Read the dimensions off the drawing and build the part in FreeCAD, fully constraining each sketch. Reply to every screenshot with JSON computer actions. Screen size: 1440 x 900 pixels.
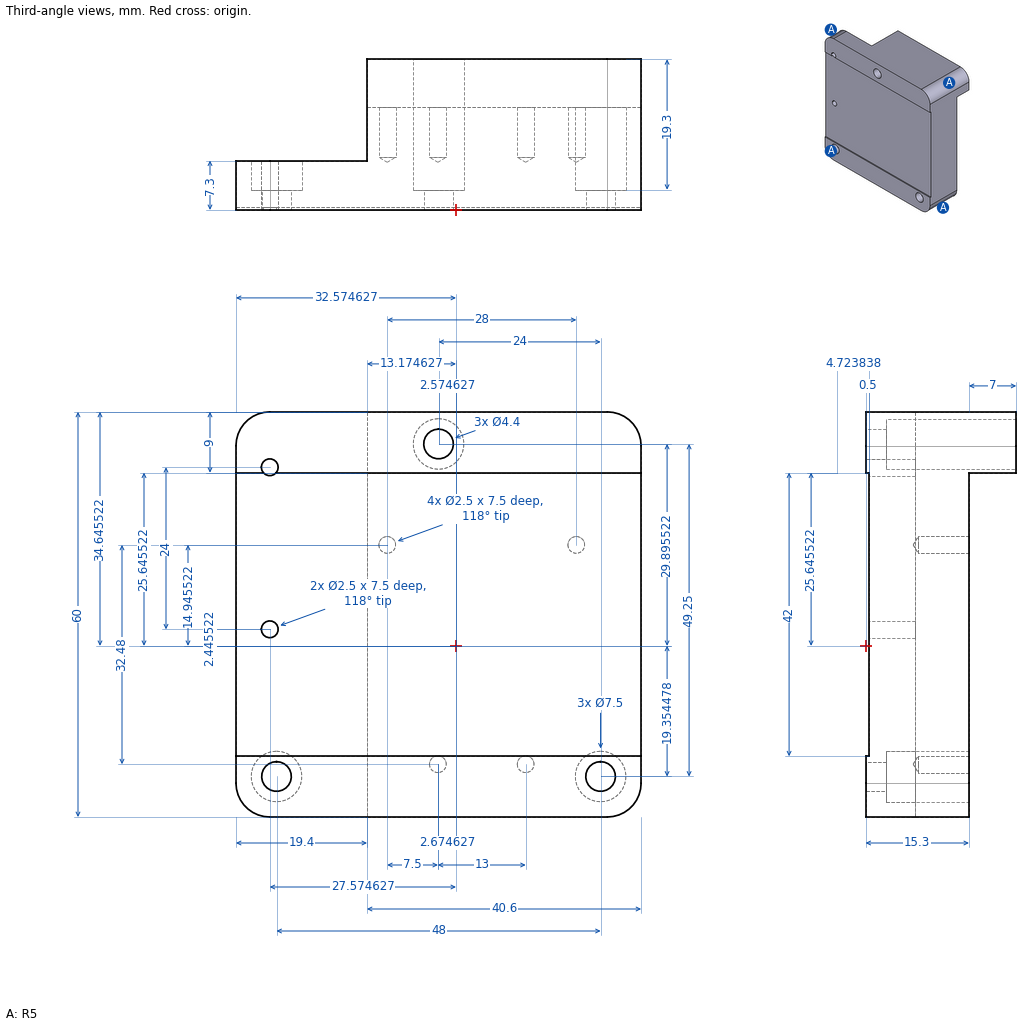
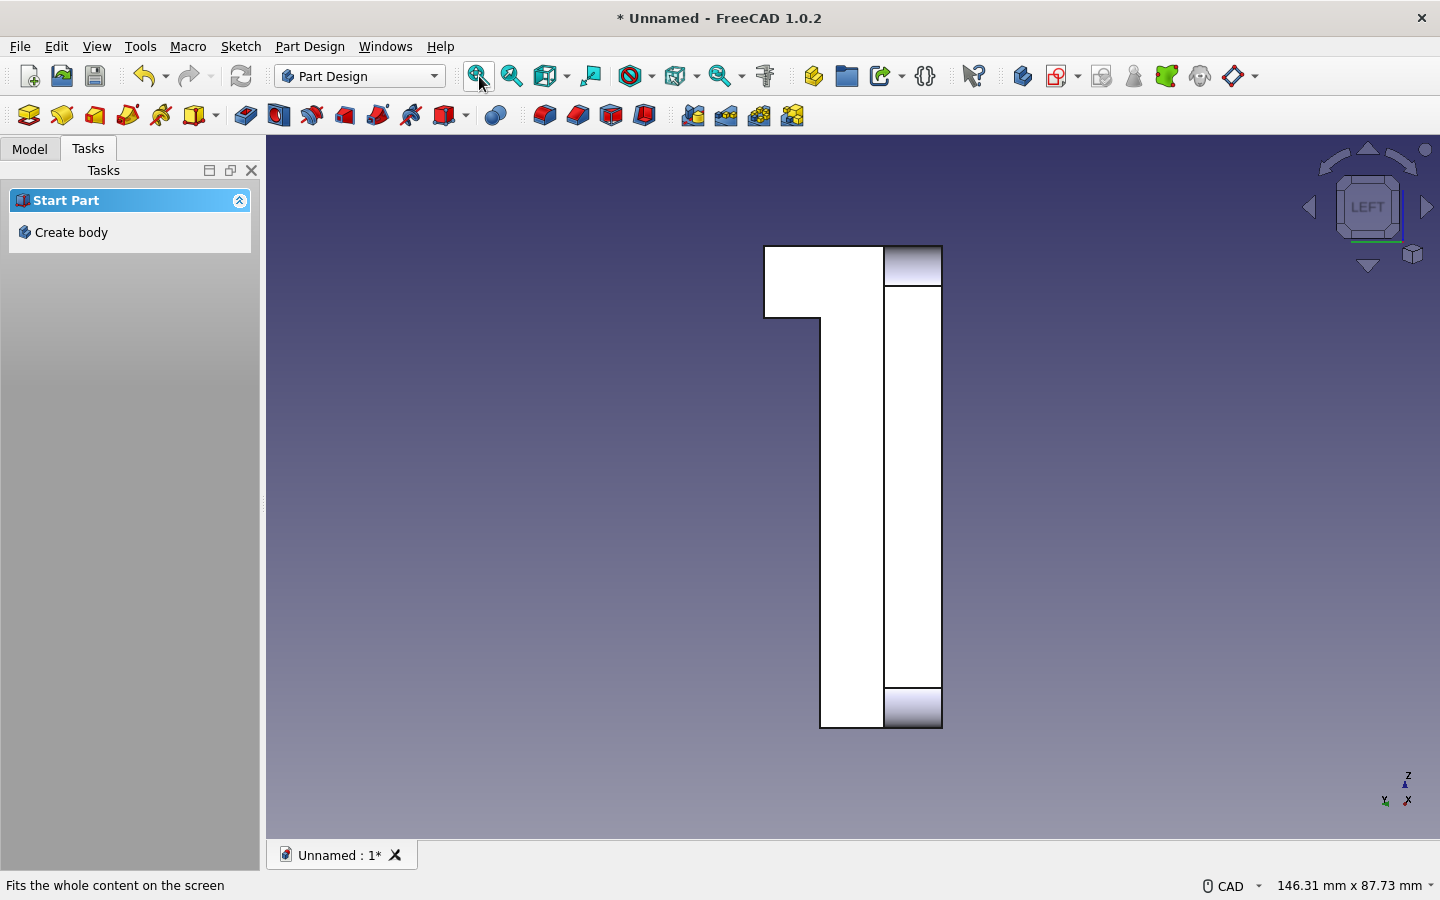
{"action": "left_click", "coordinate": [913, 543]}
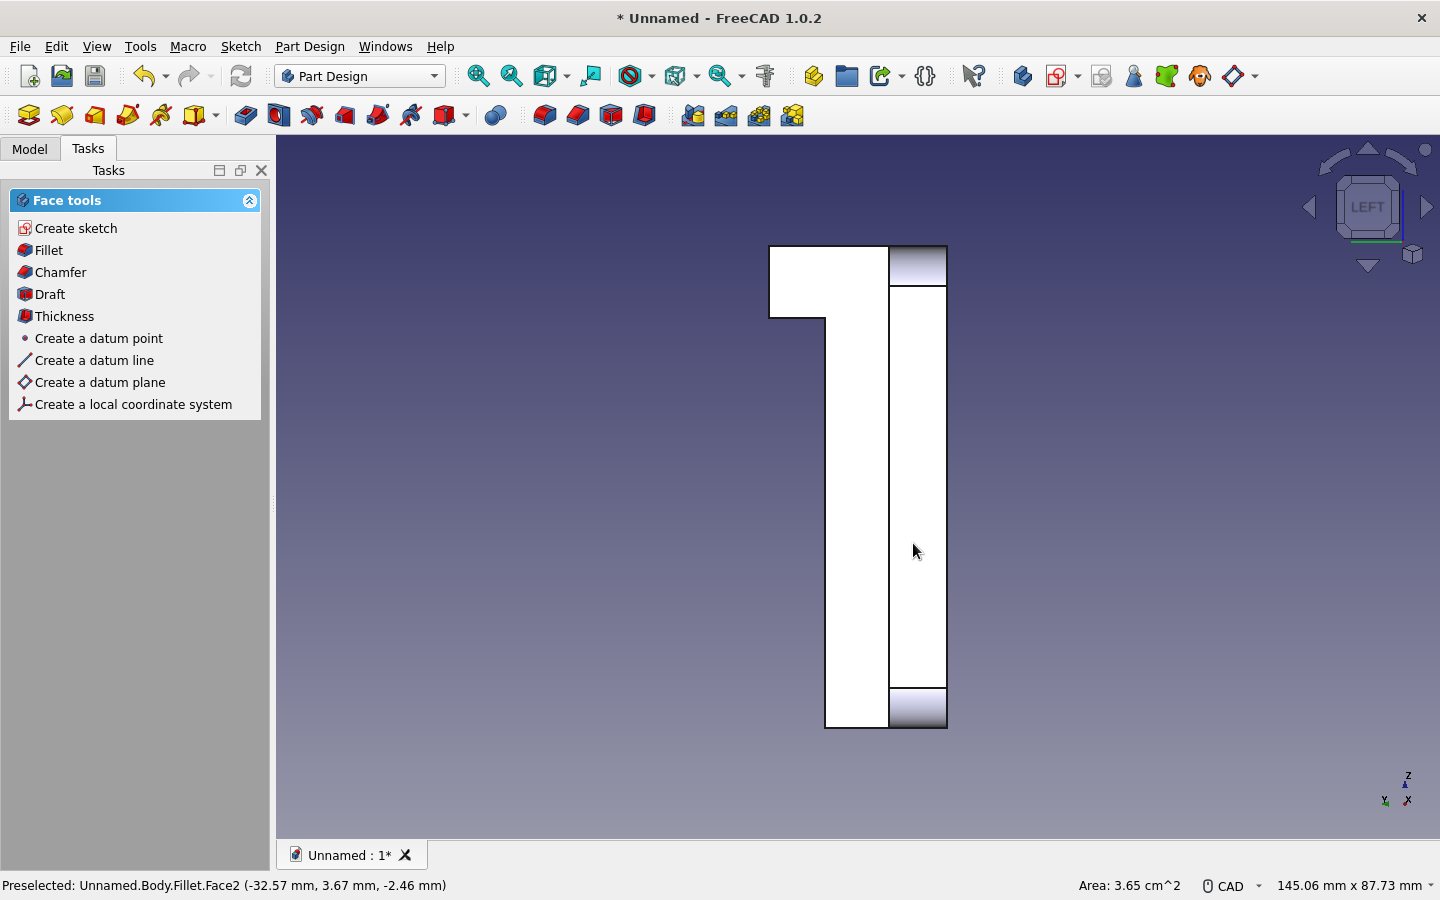
{"action": "left_click", "coordinate": [1056, 76]}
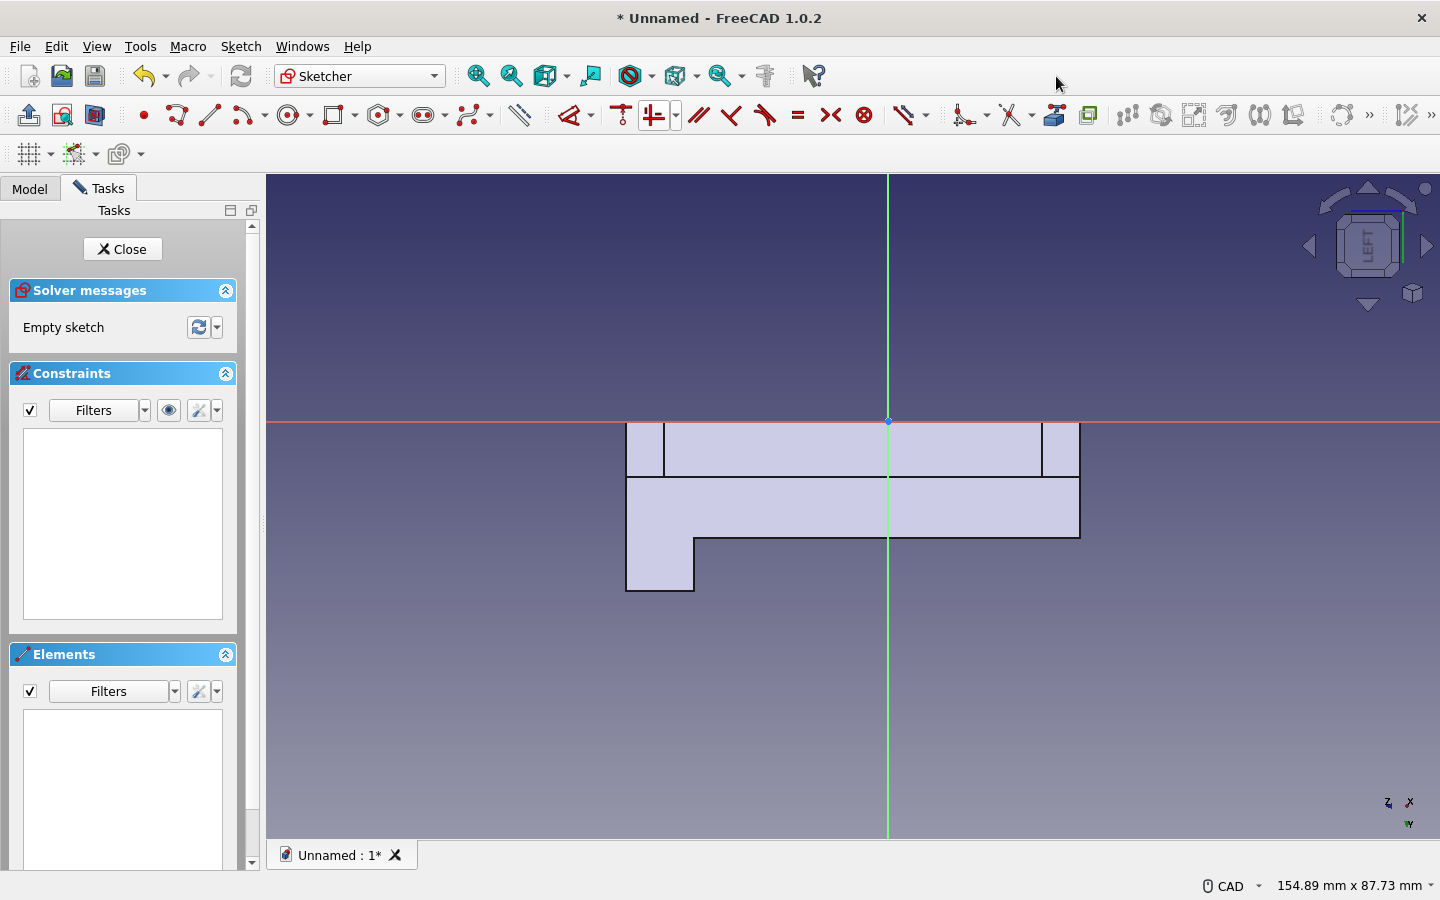
{"action": "scroll", "coordinate": [909, 327], "scroll_direction": "up", "scroll_amount": 4}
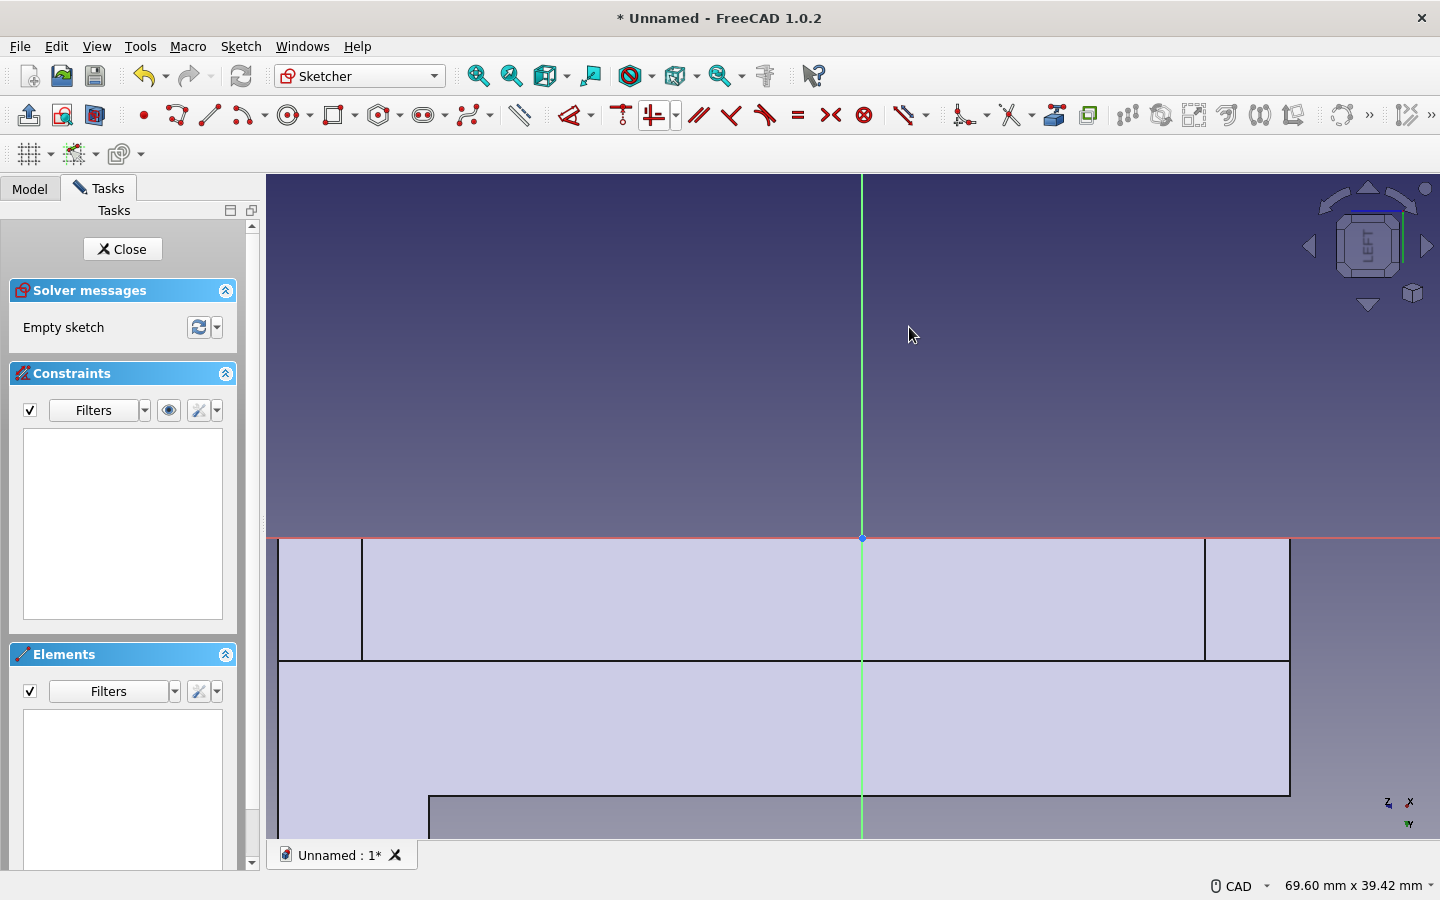
{"action": "left_click", "coordinate": [332, 116]}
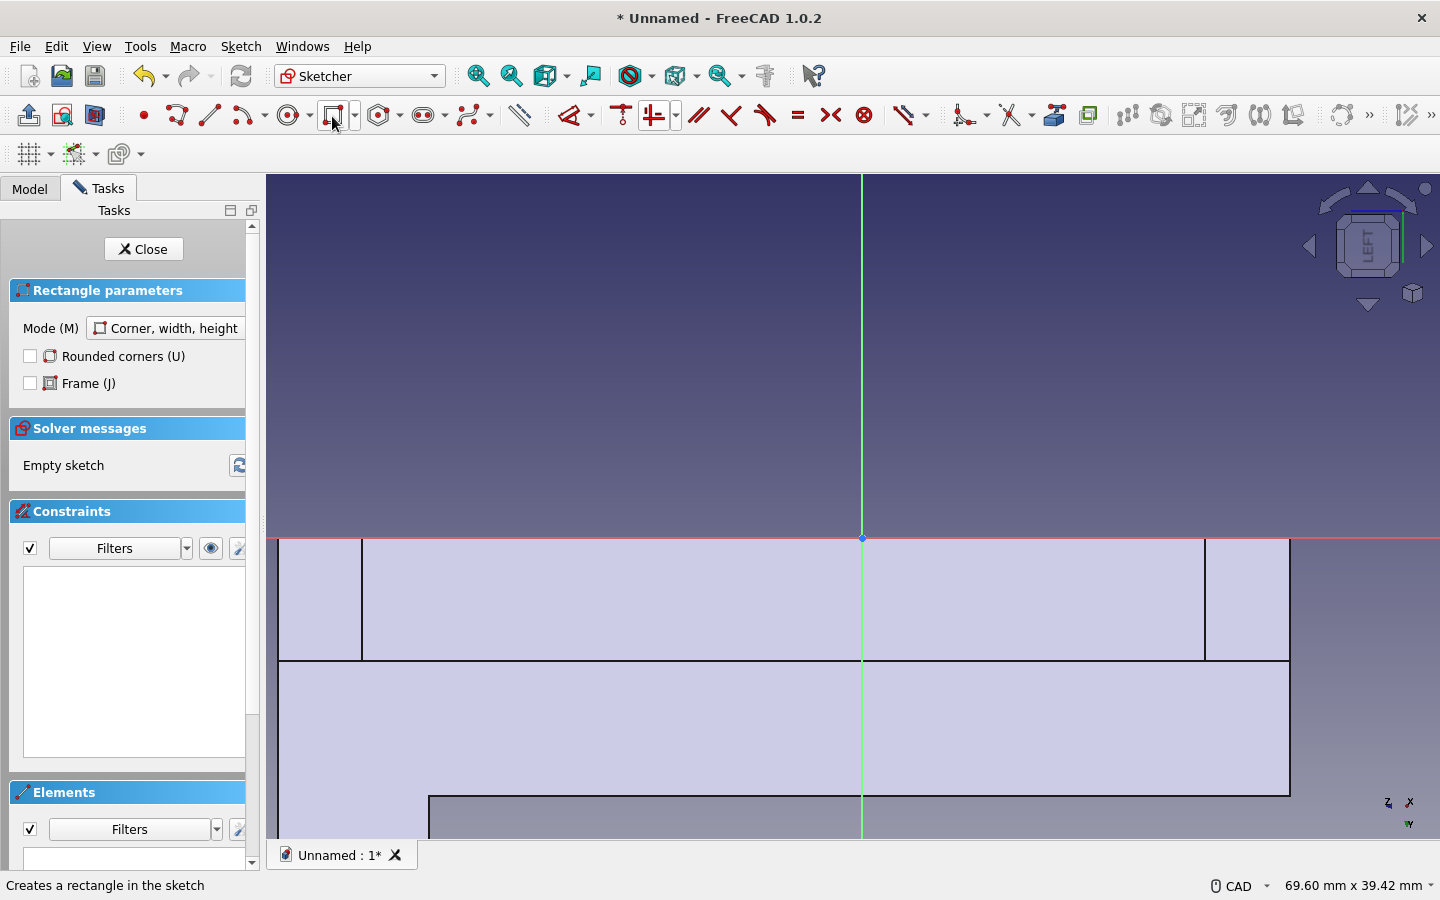
{"action": "left_click", "coordinate": [429, 467]}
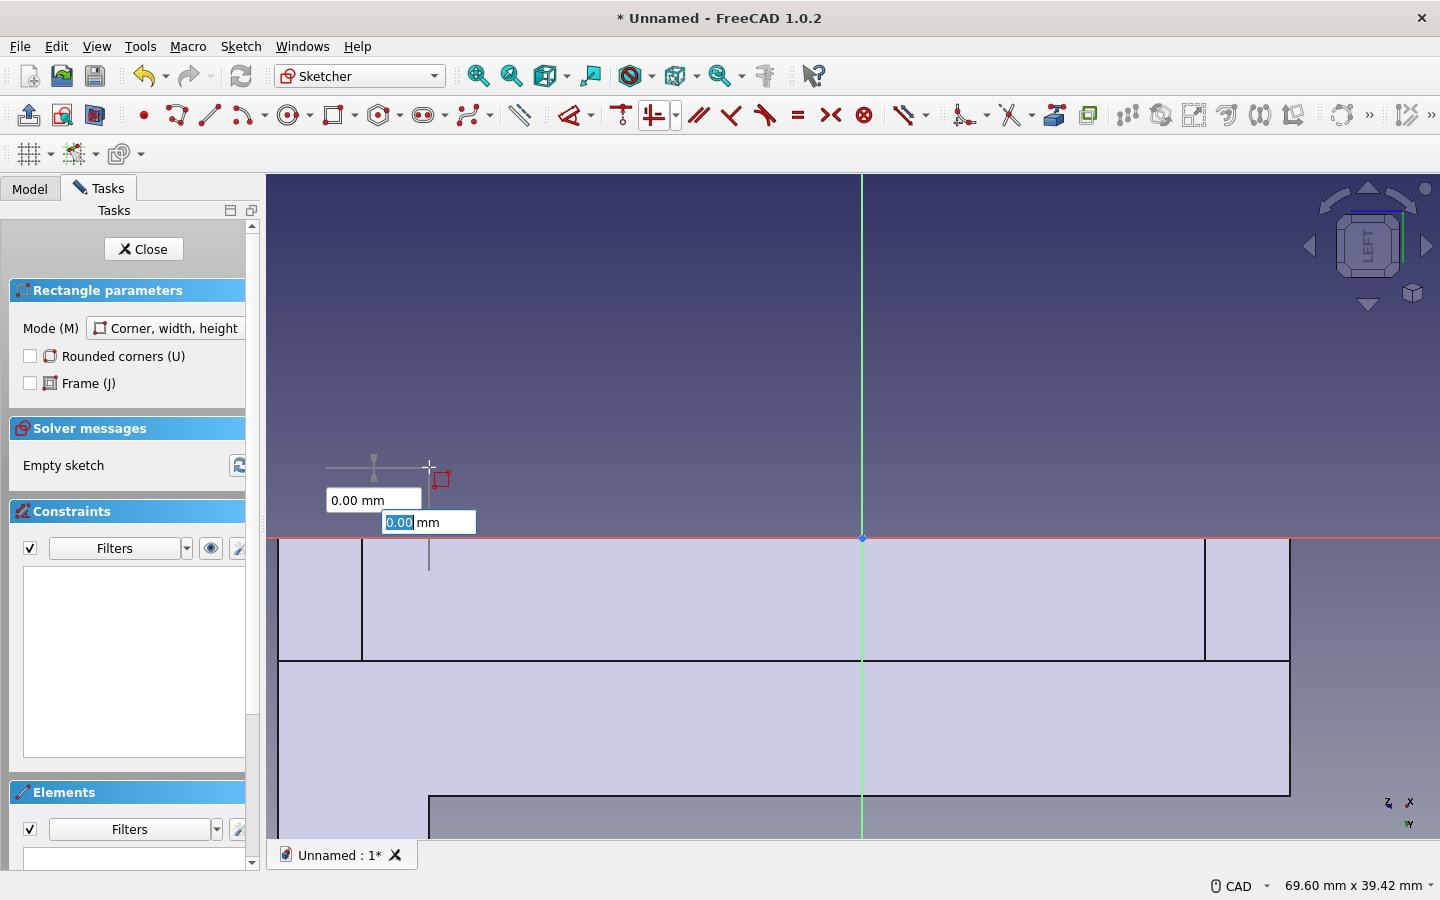
{"action": "scroll", "coordinate": [1138, 547], "scroll_direction": "up", "scroll_amount": 4}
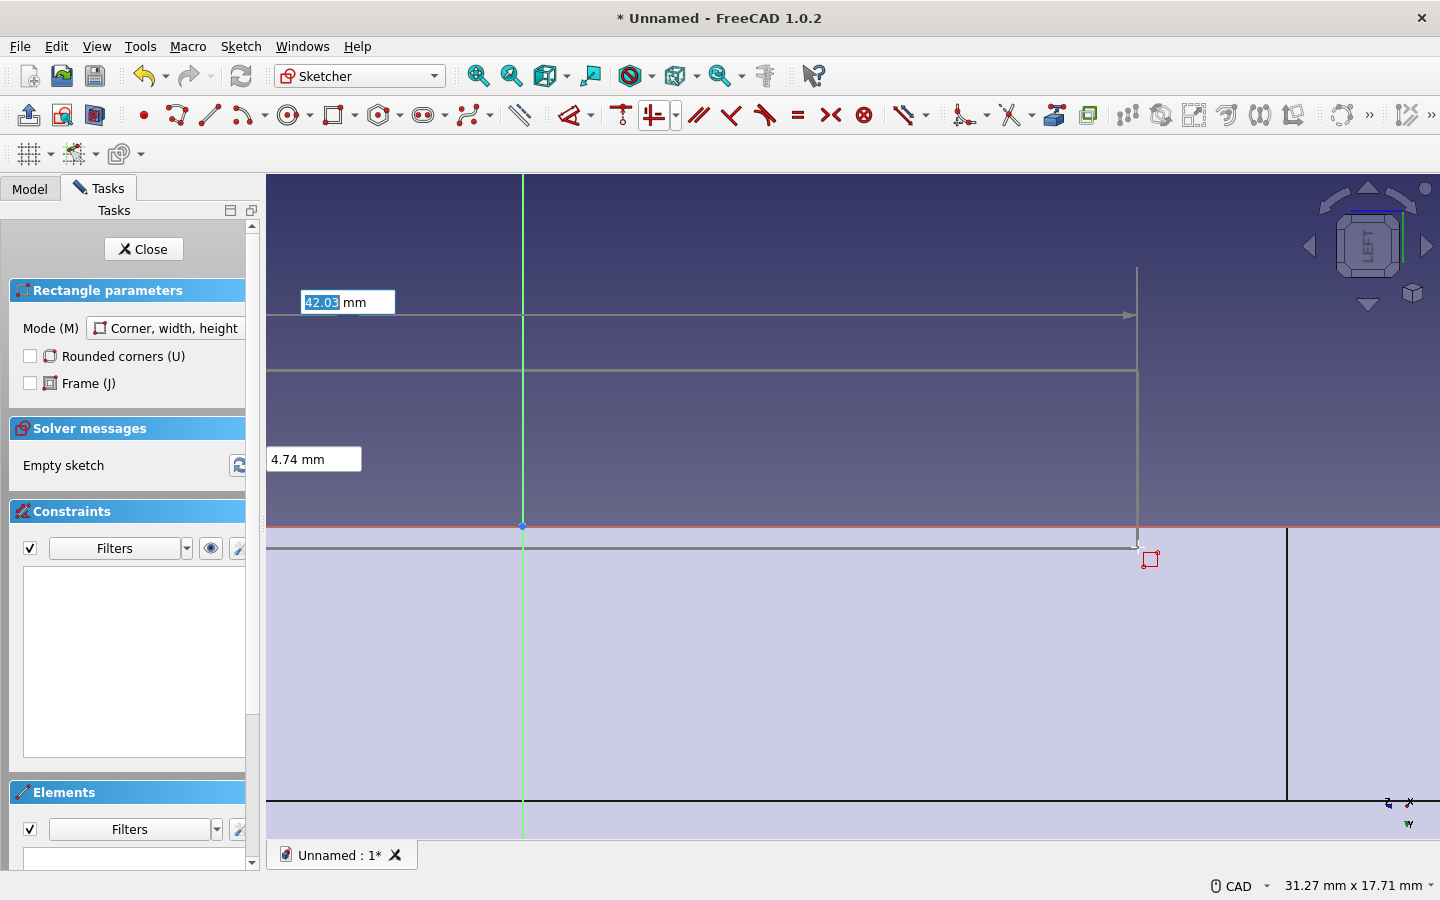
{"action": "left_click", "coordinate": [1137, 545]}
{"action": "key", "text": "Escape"}